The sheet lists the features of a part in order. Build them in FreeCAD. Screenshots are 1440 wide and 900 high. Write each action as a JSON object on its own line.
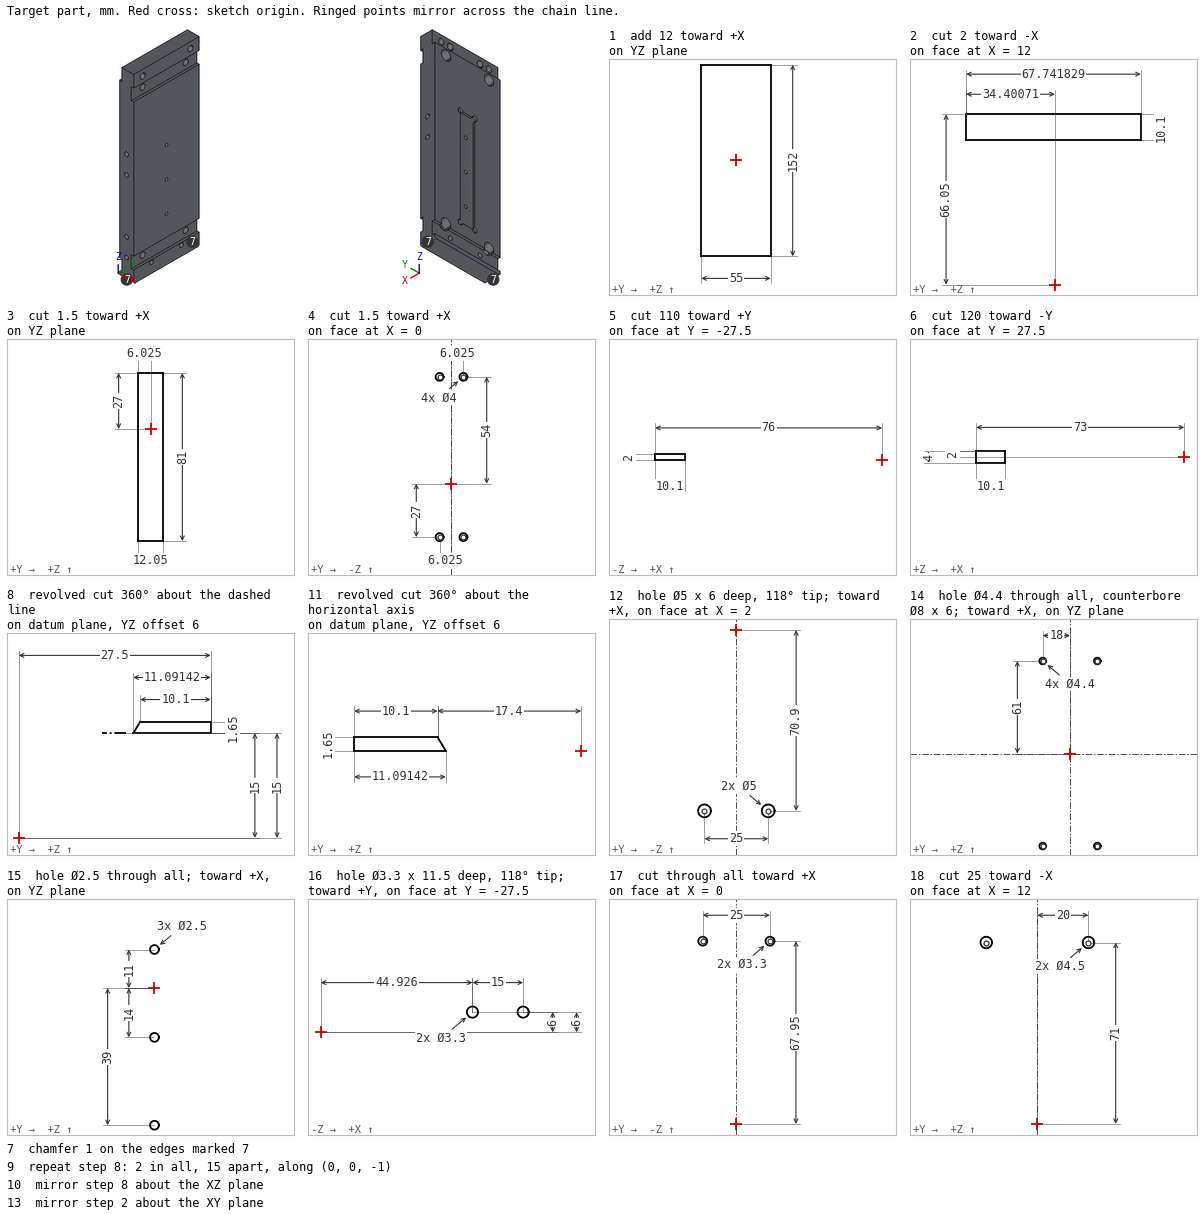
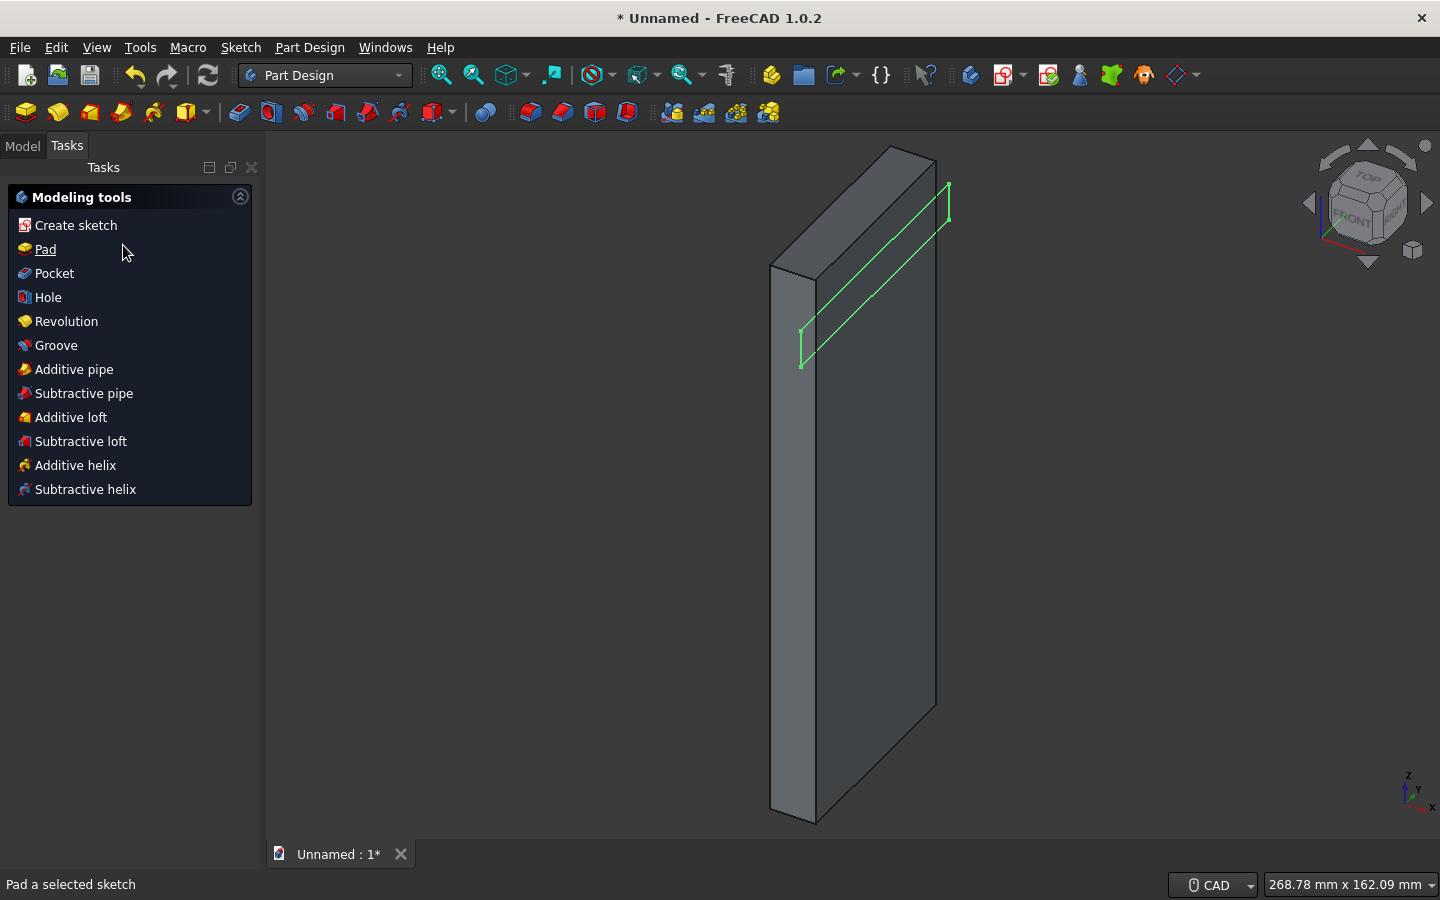
{"action": "left_click", "coordinate": [240, 112]}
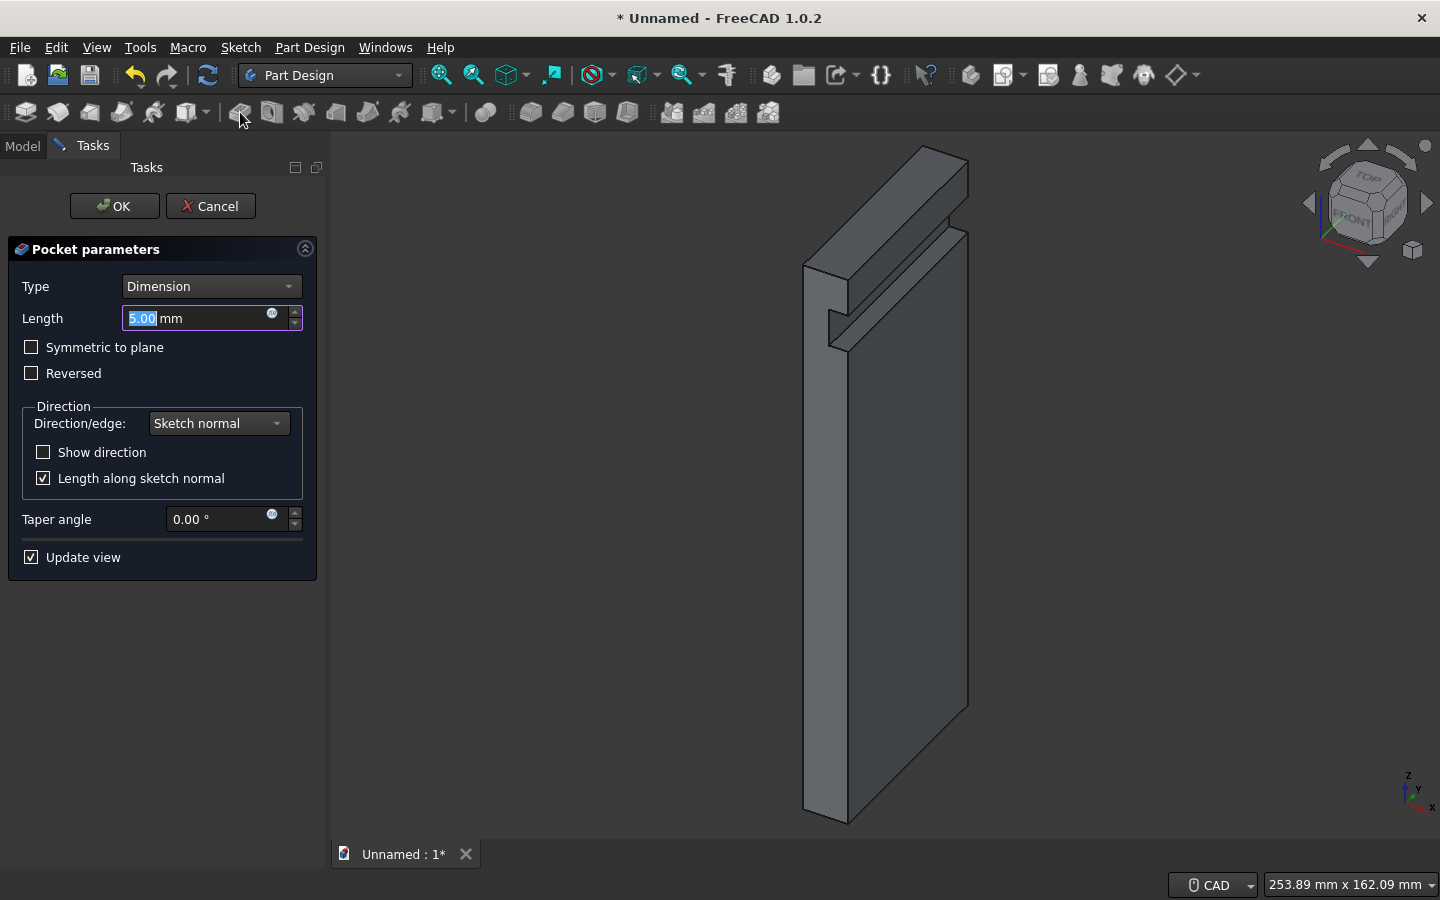
{"action": "type", "text": "2"}
{"action": "key", "text": "Tab"}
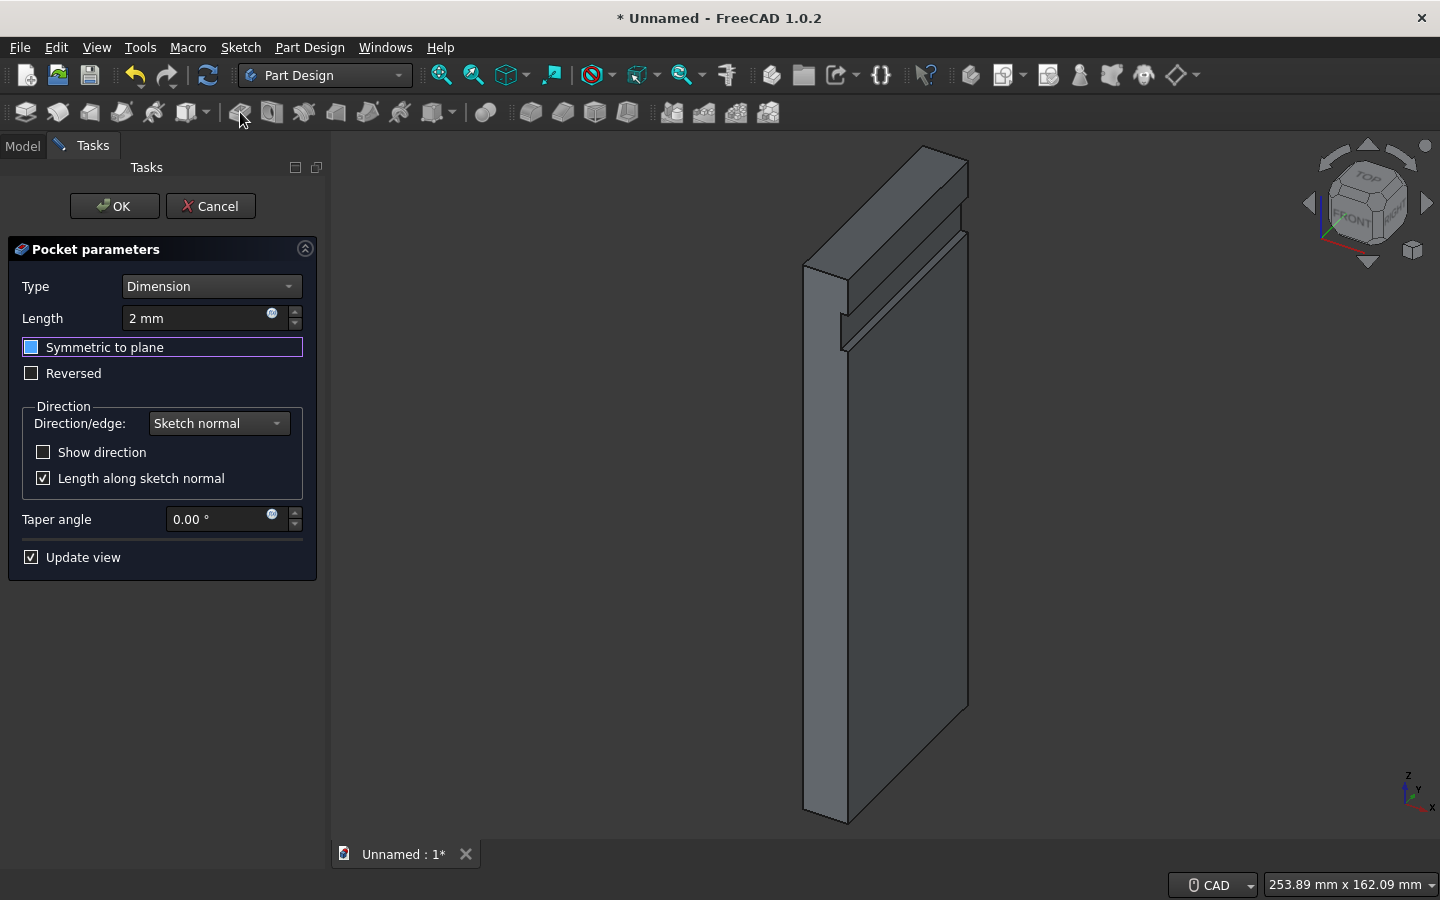
{"action": "left_click", "coordinate": [115, 206]}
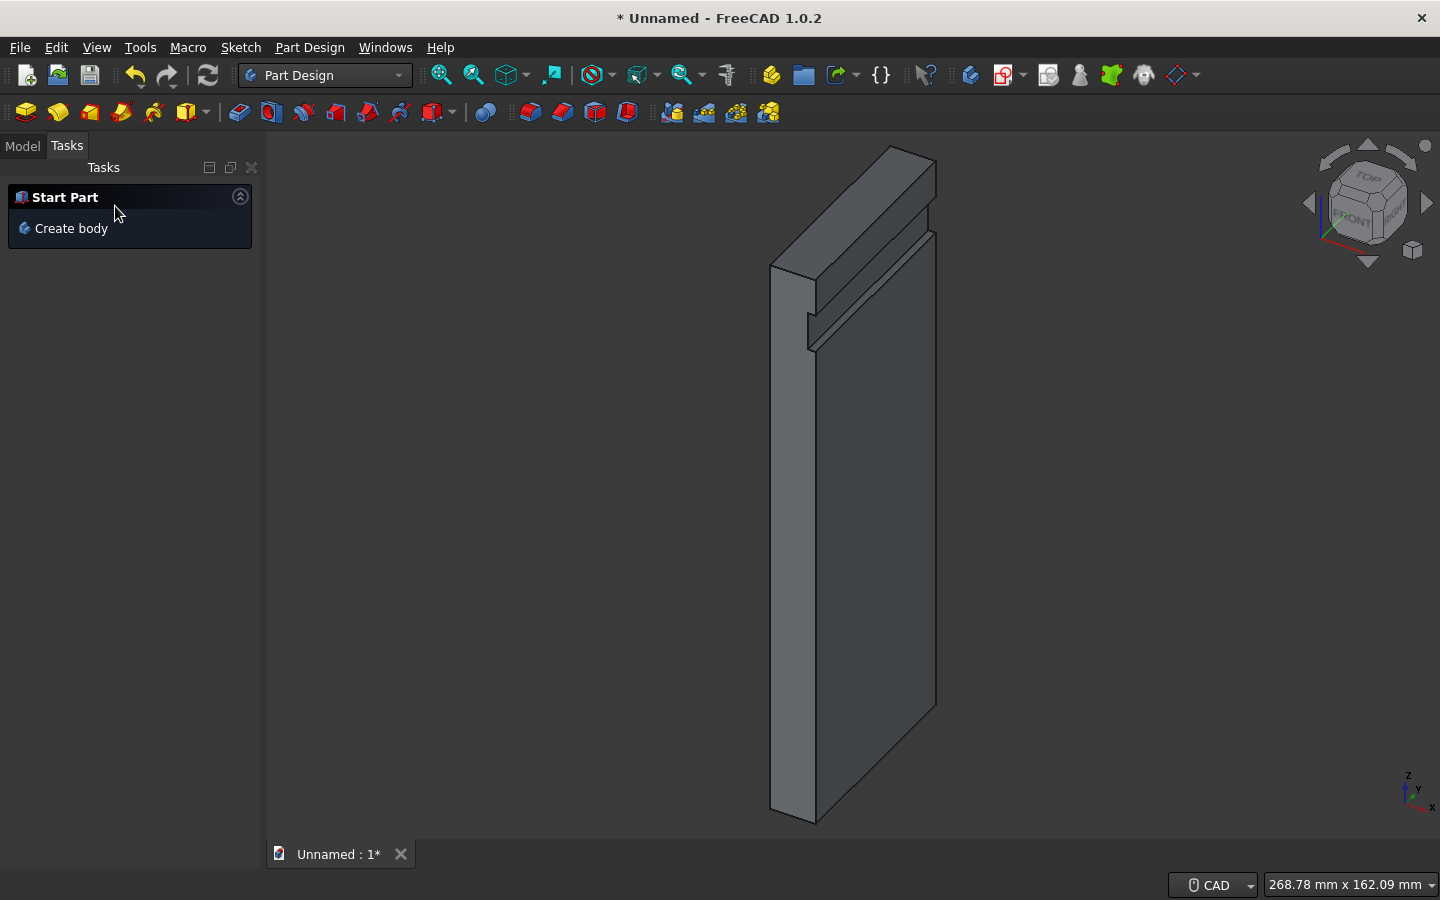
{"action": "left_click", "coordinate": [1004, 76]}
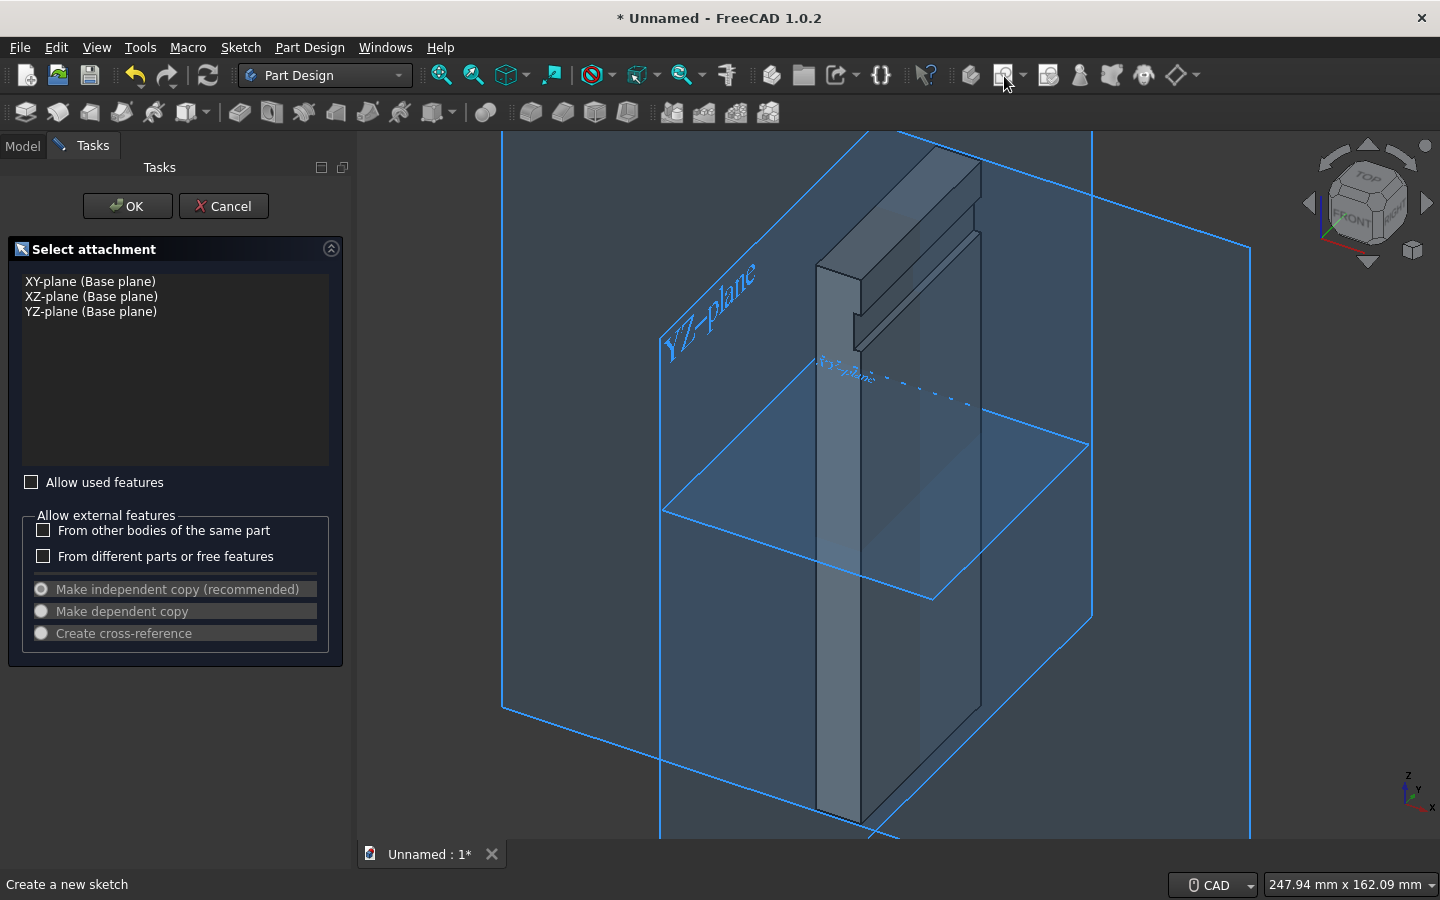
{"action": "left_click", "coordinate": [82, 312]}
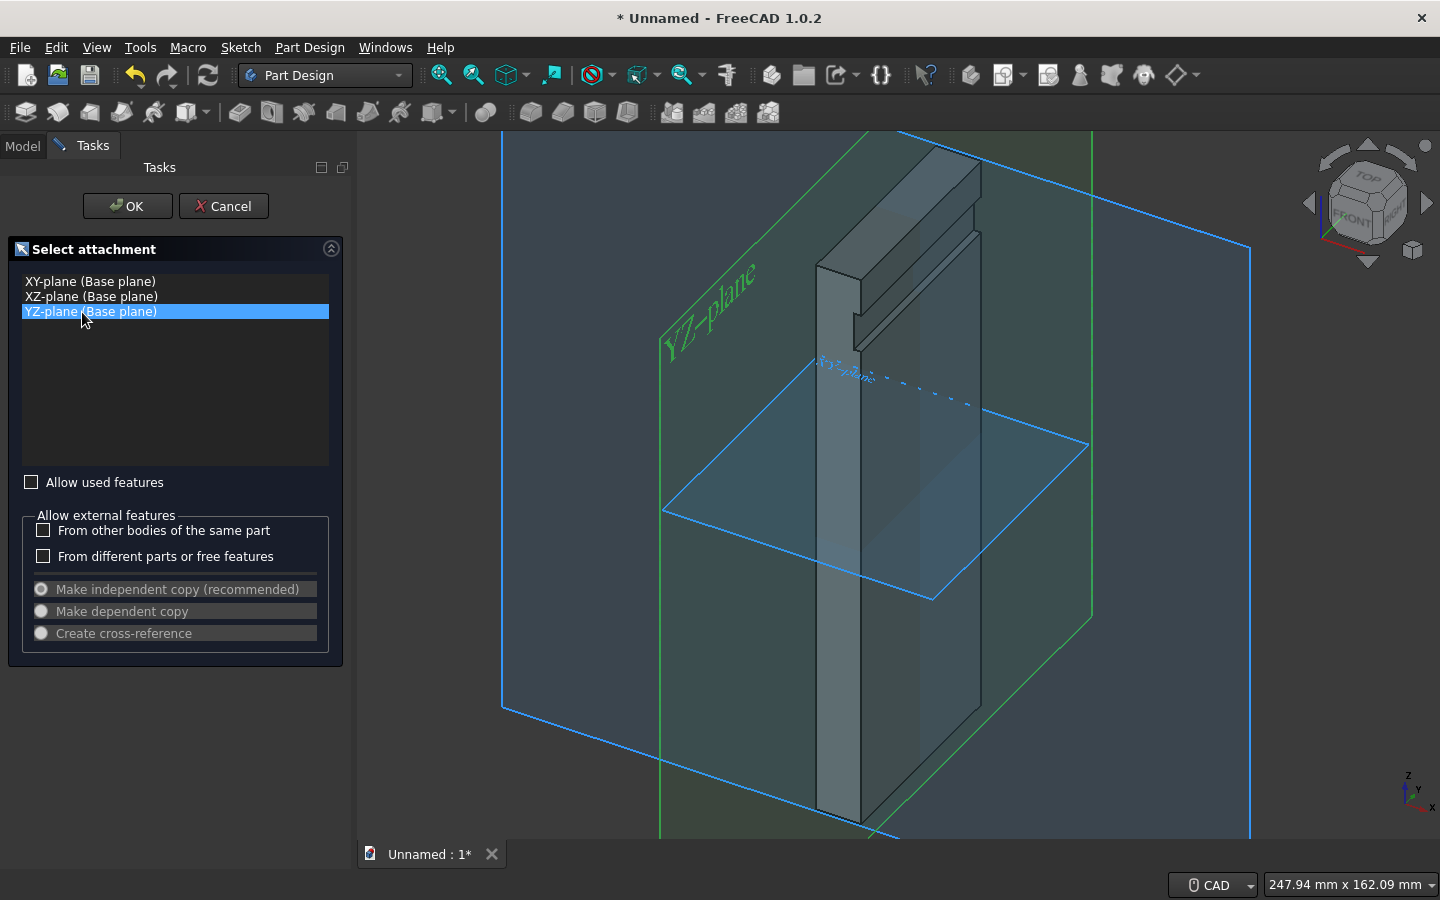
{"action": "left_click", "coordinate": [128, 206]}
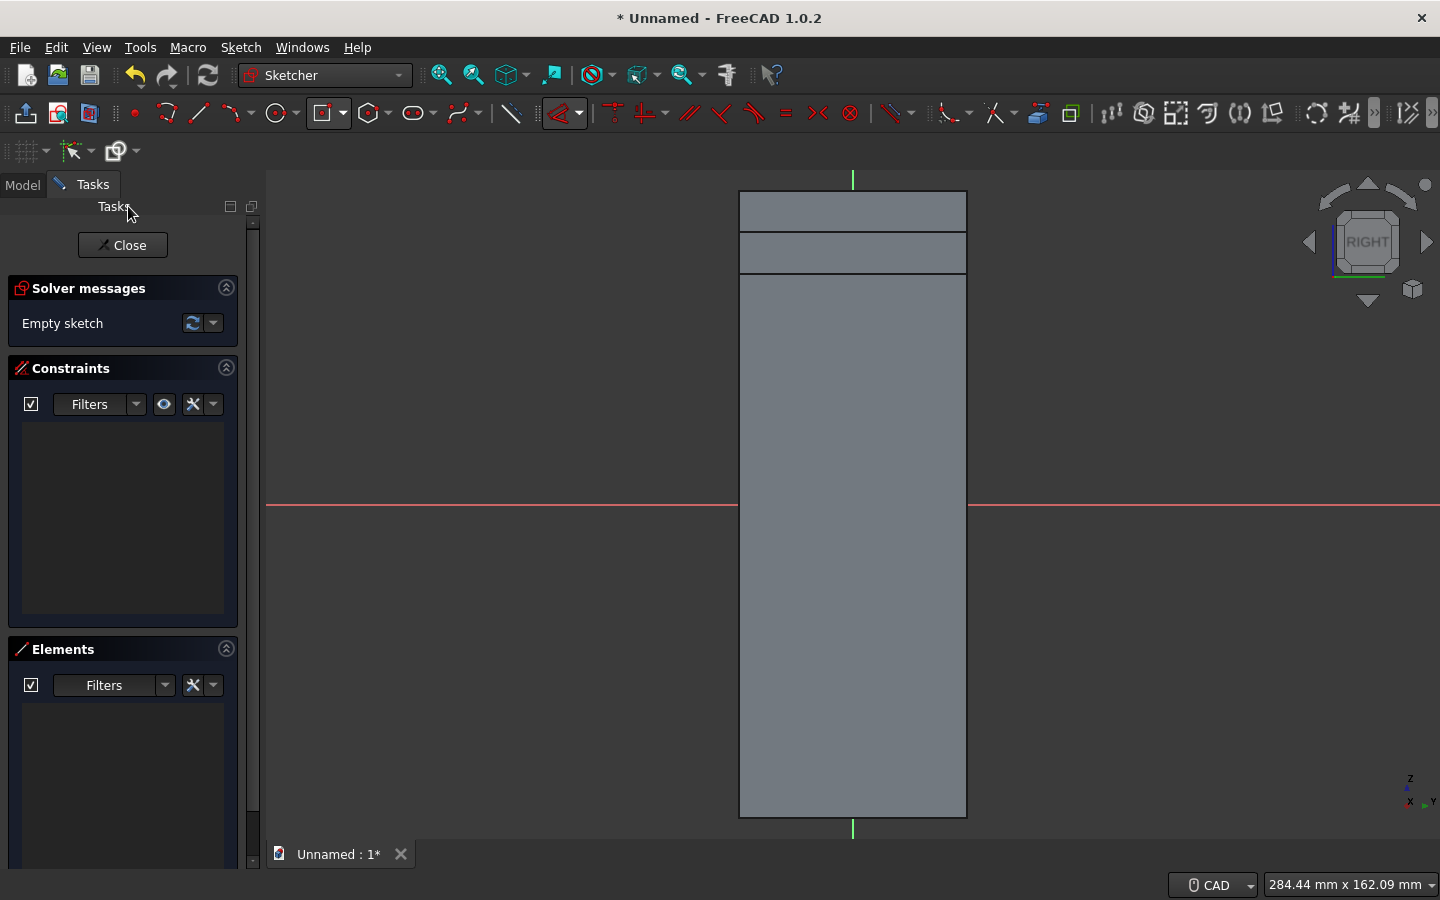
{"action": "left_click", "coordinate": [90, 114]}